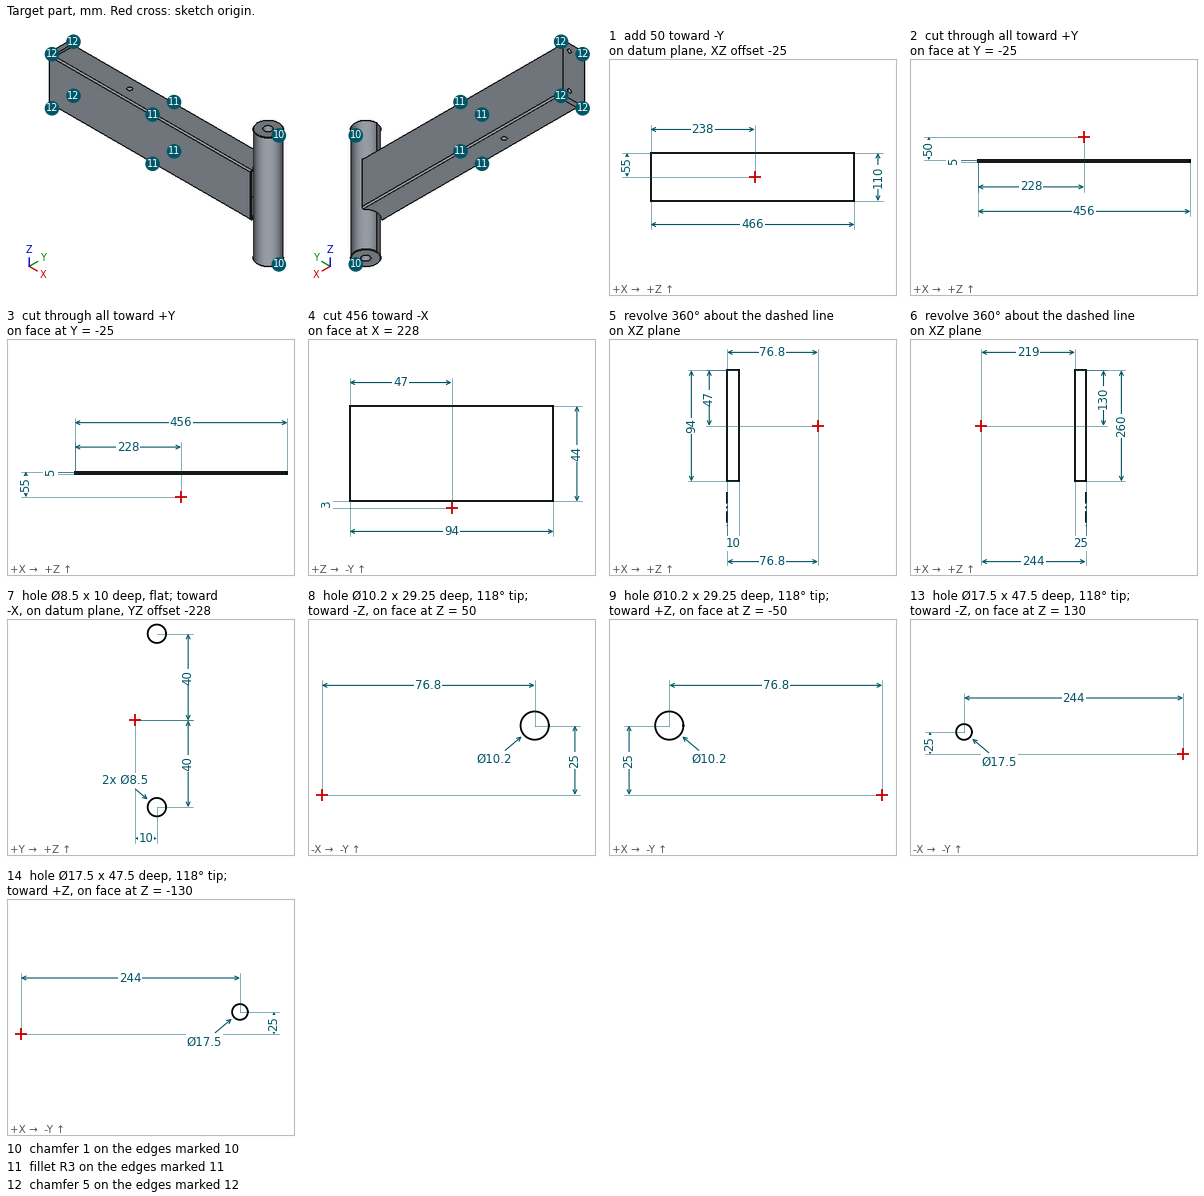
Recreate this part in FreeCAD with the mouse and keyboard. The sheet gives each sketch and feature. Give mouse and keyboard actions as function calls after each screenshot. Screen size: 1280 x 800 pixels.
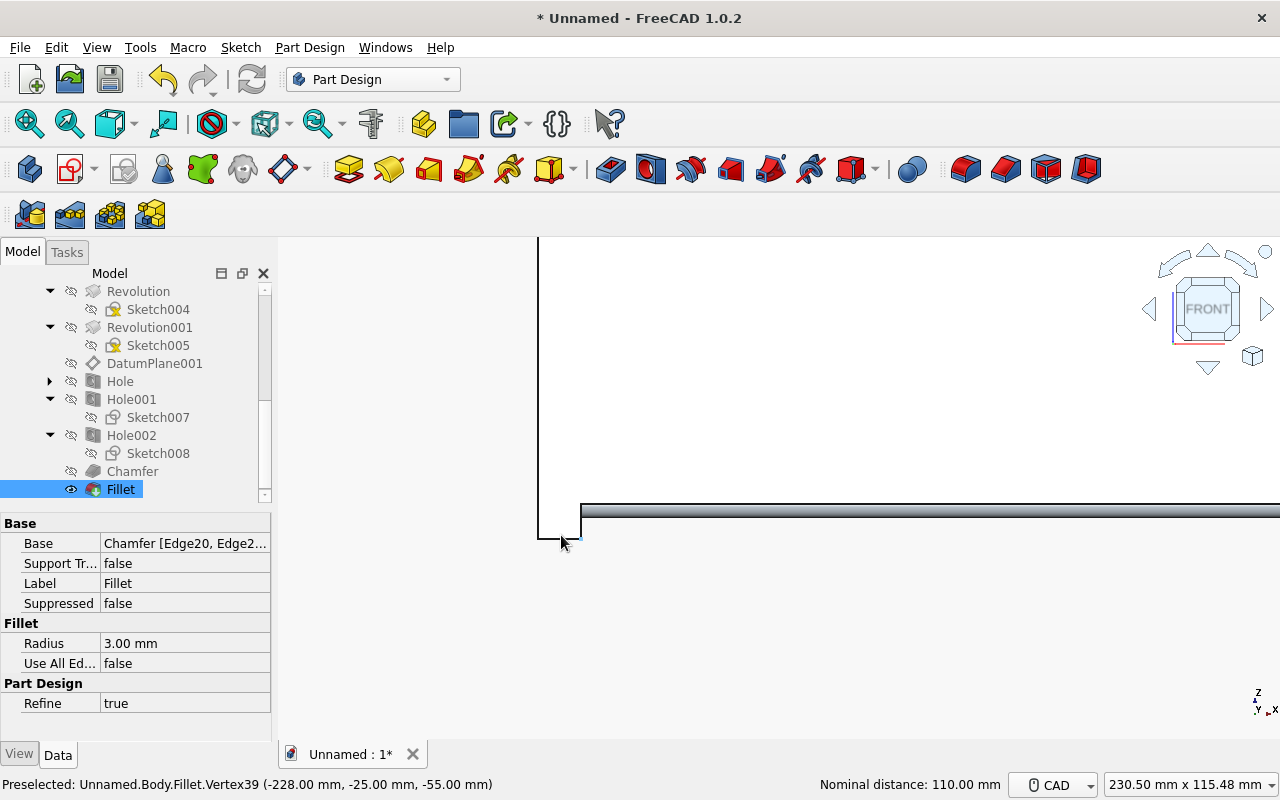
click(30, 124)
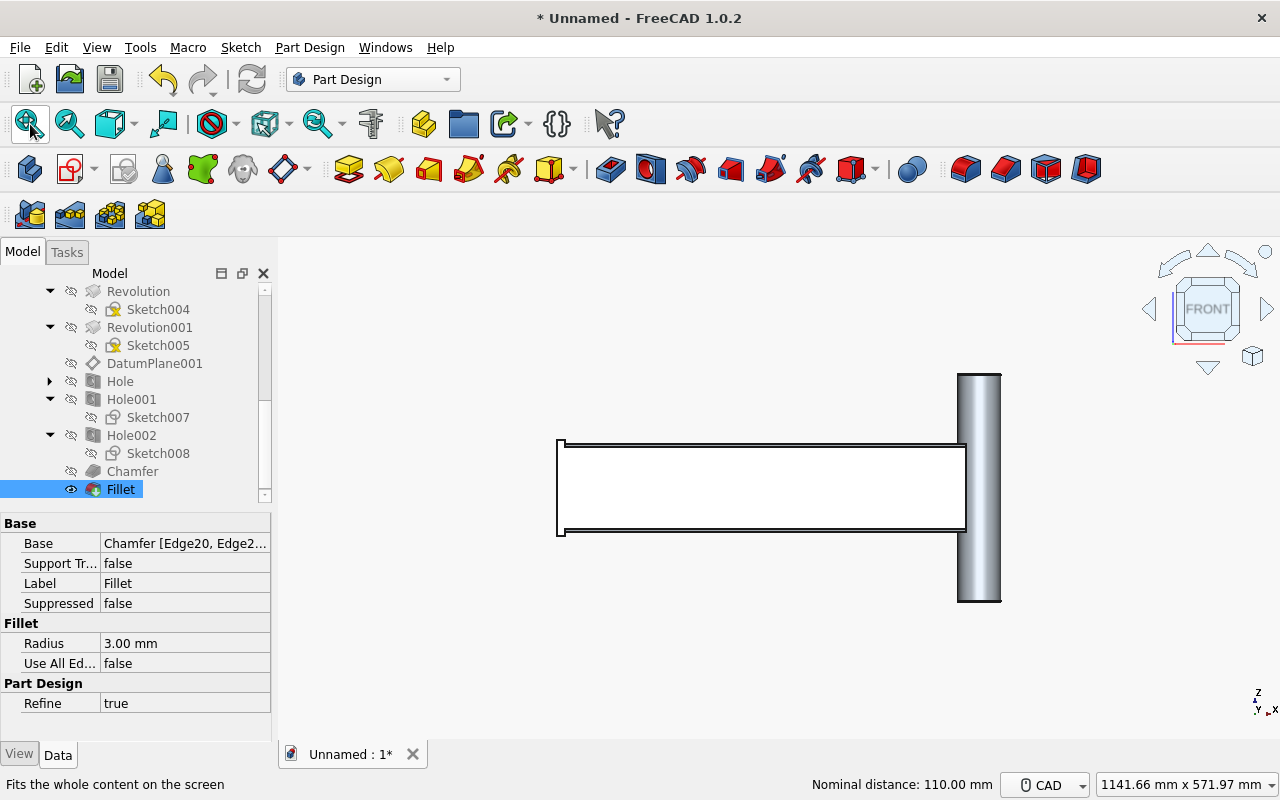
key(3)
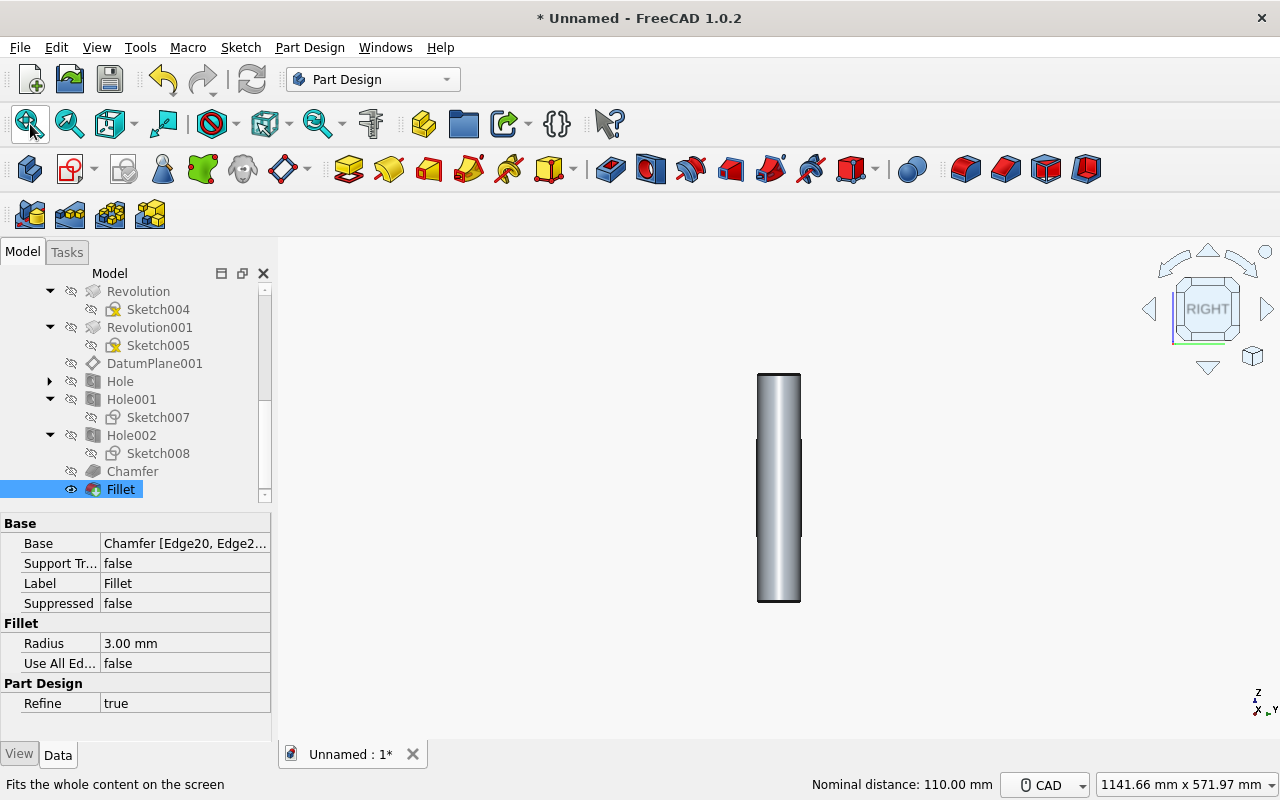
scroll(757, 535, up, 8)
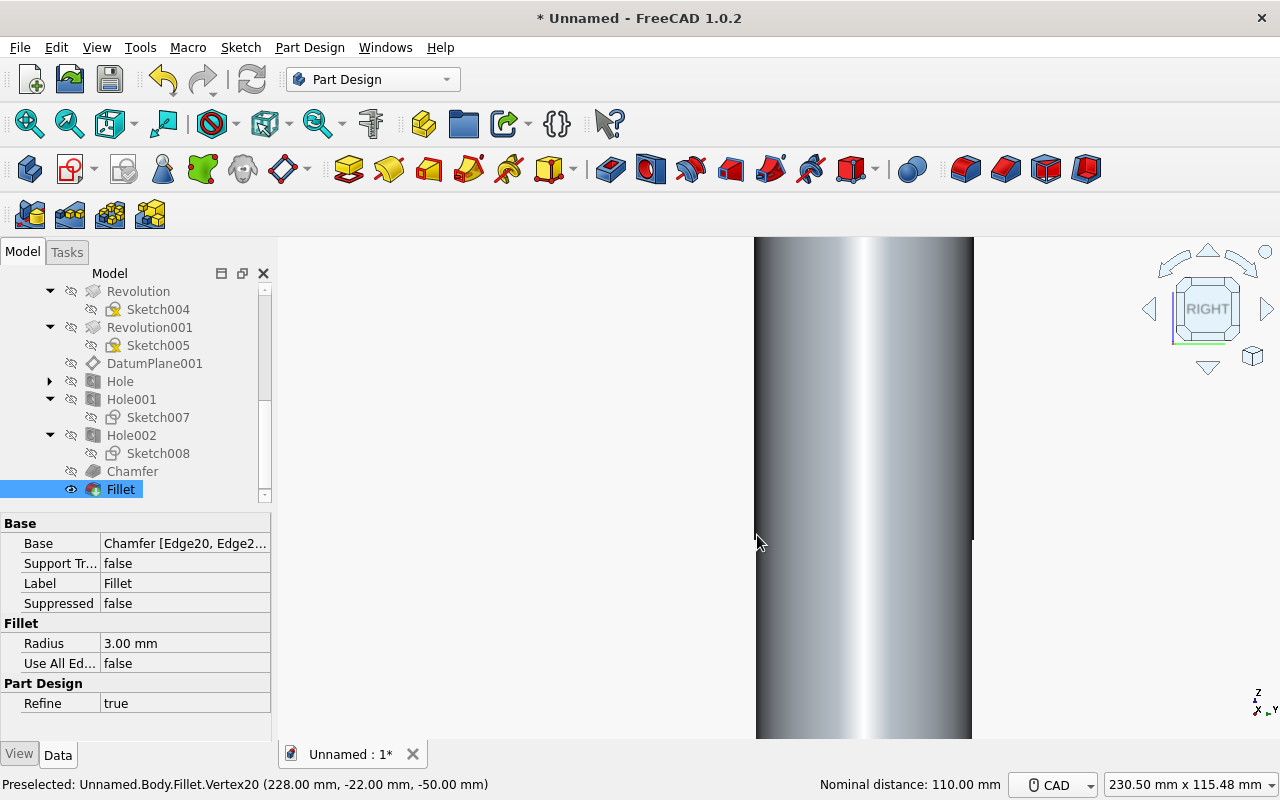
click(30, 124)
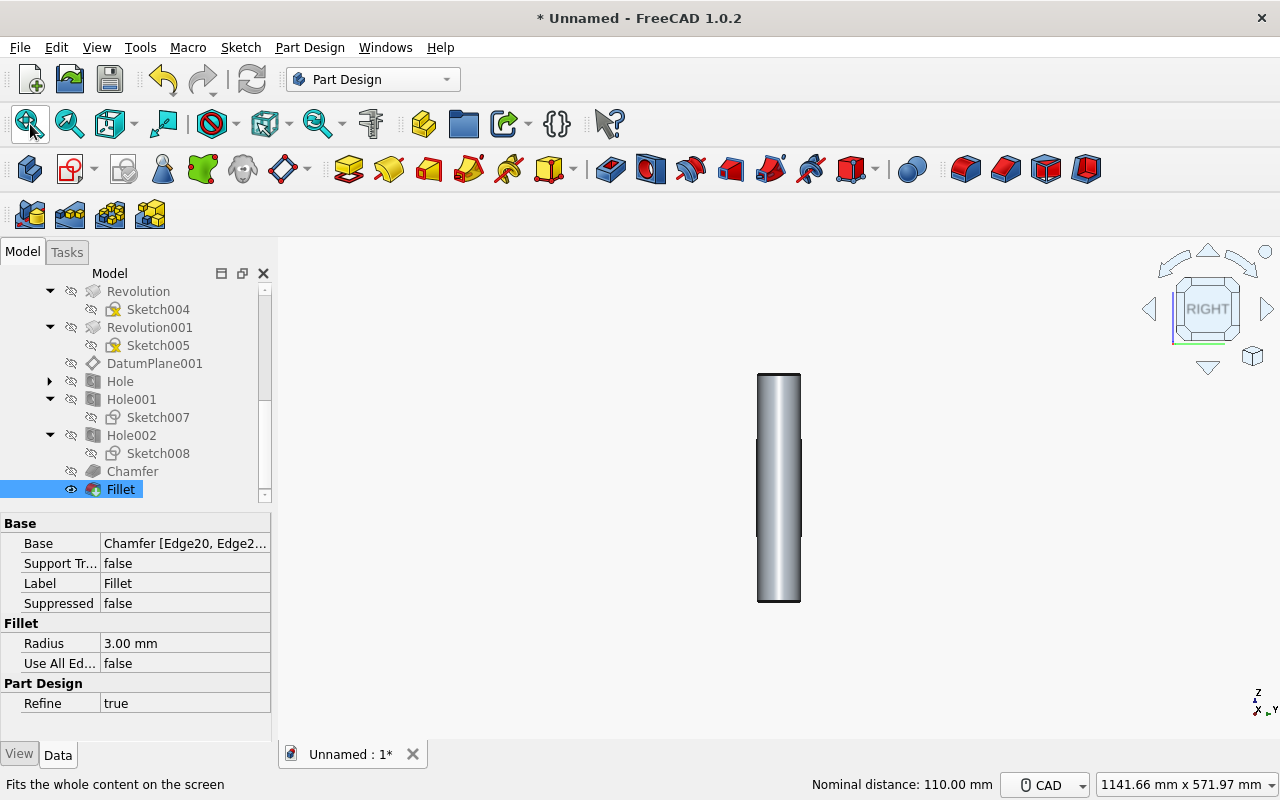
key(5)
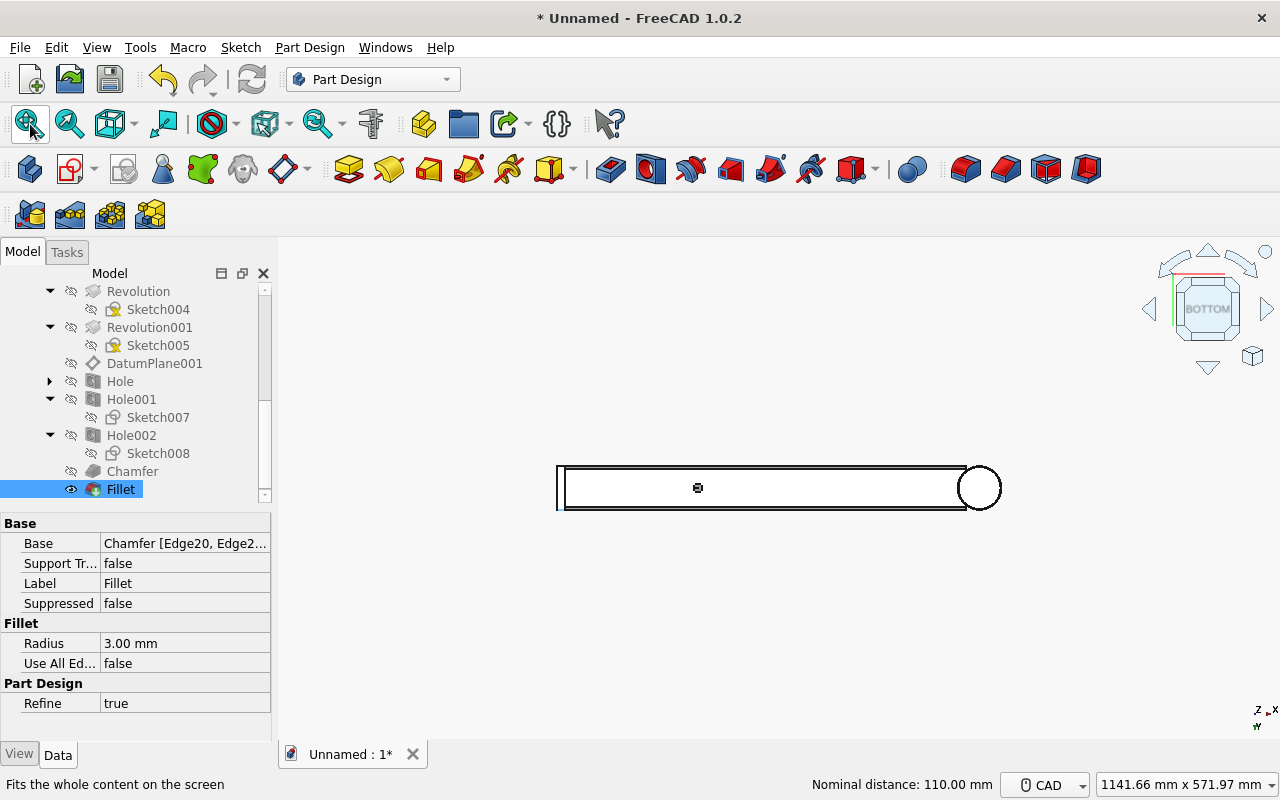
click(30, 124)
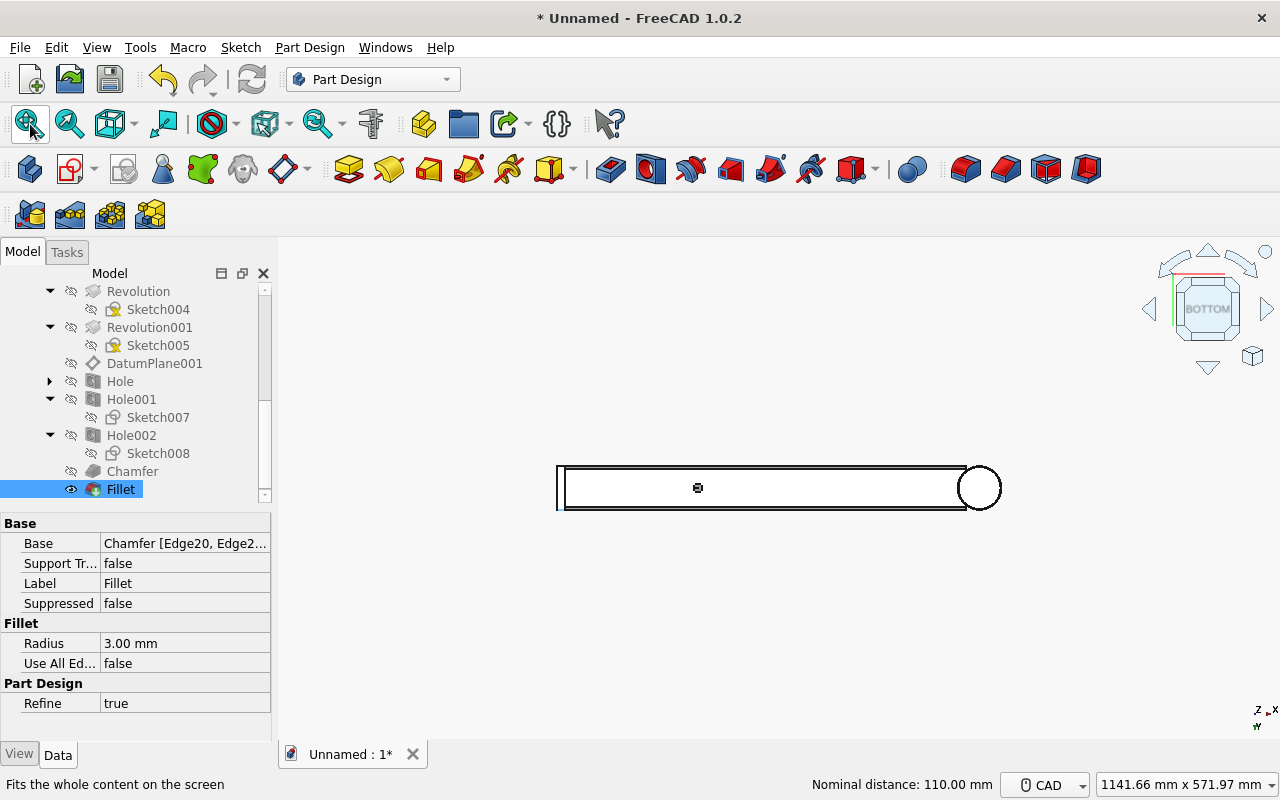
scroll(561, 465, up, 8)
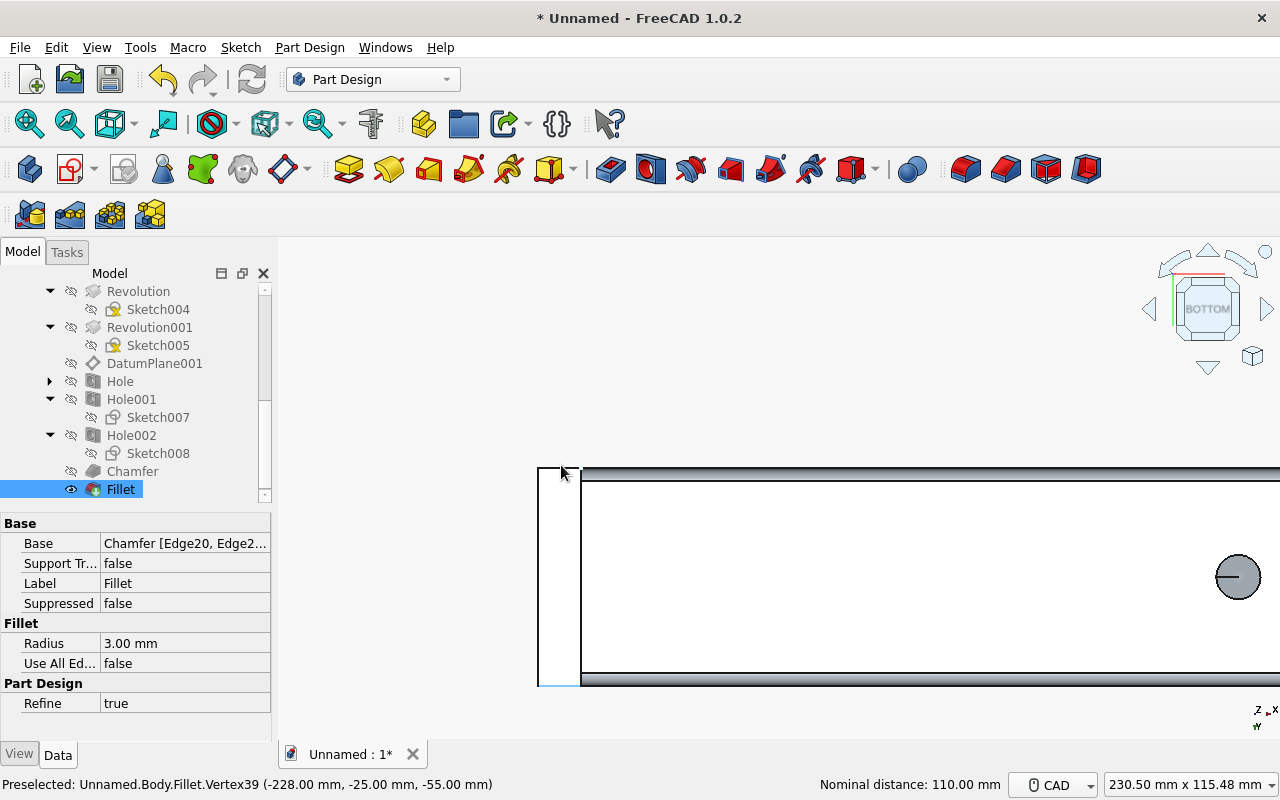
click(559, 467, ctrl)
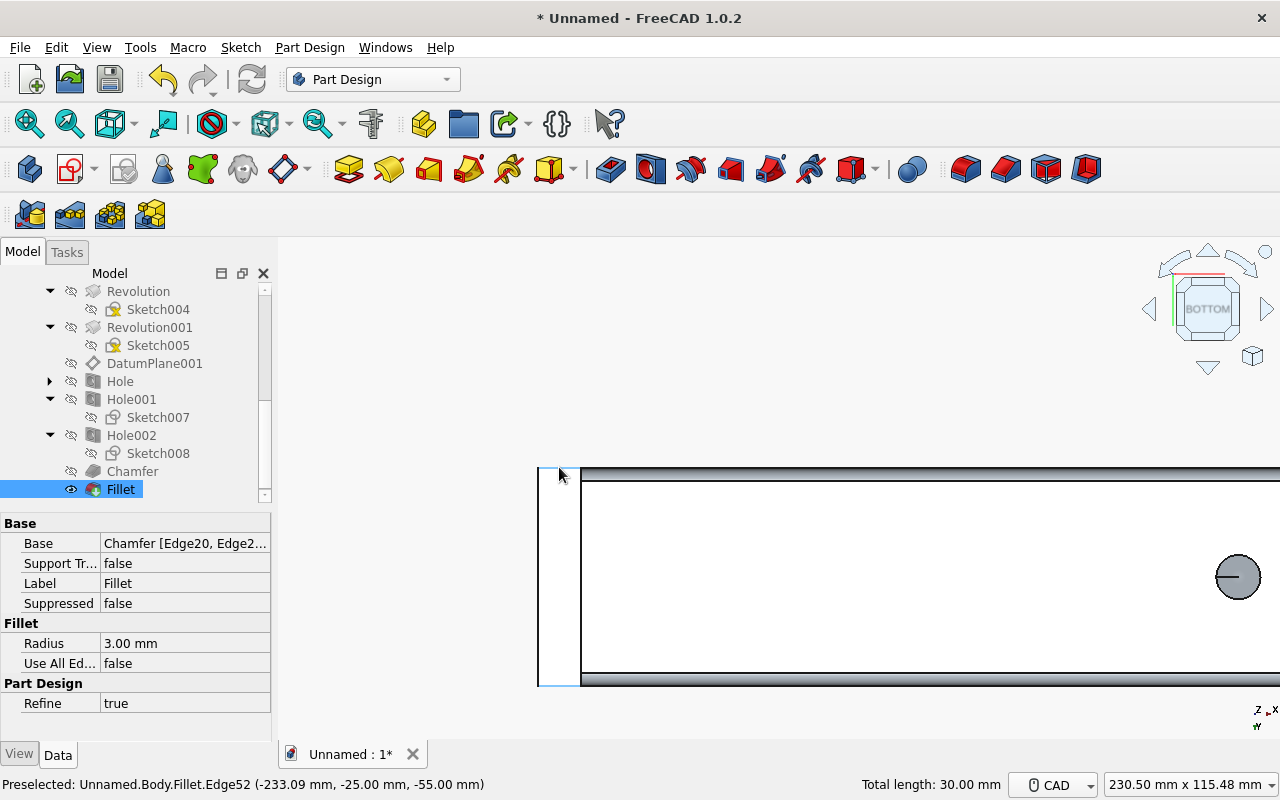
click(30, 124)